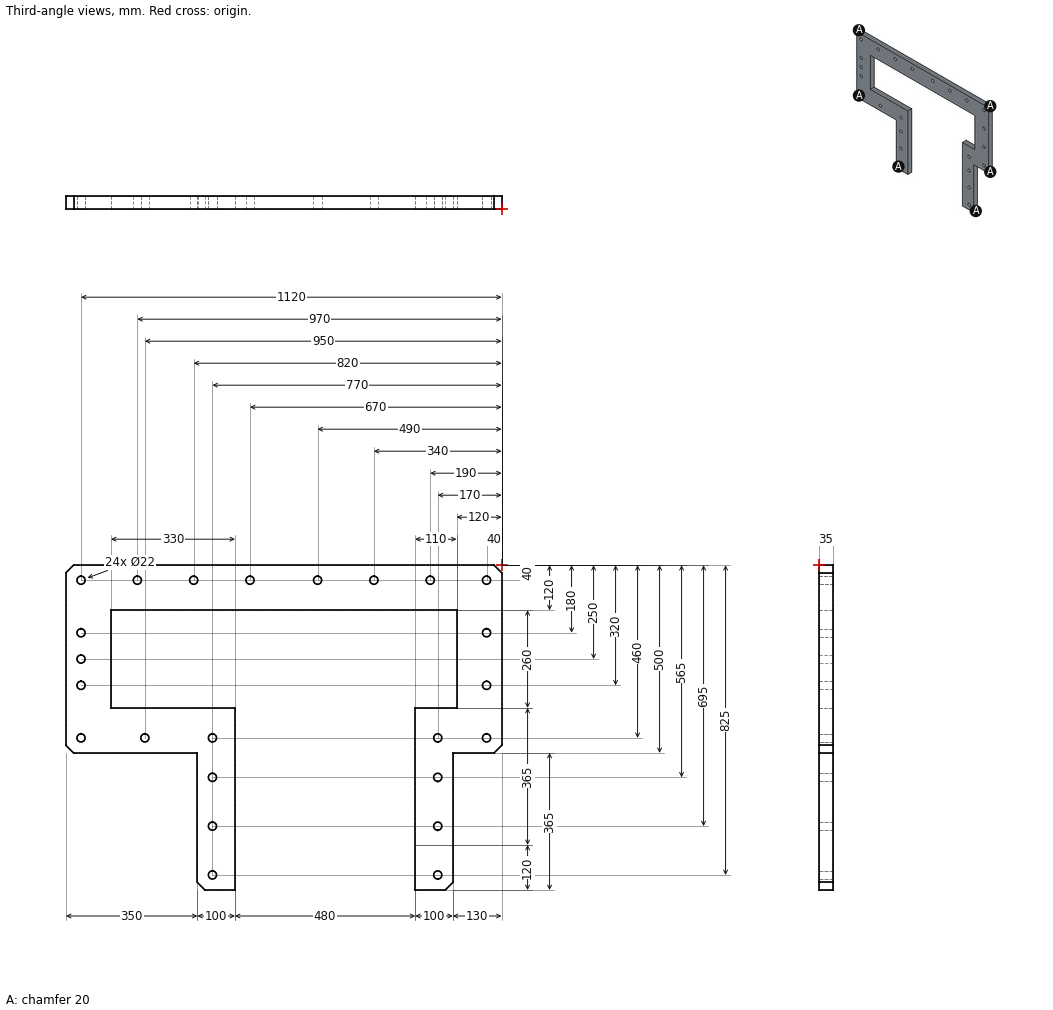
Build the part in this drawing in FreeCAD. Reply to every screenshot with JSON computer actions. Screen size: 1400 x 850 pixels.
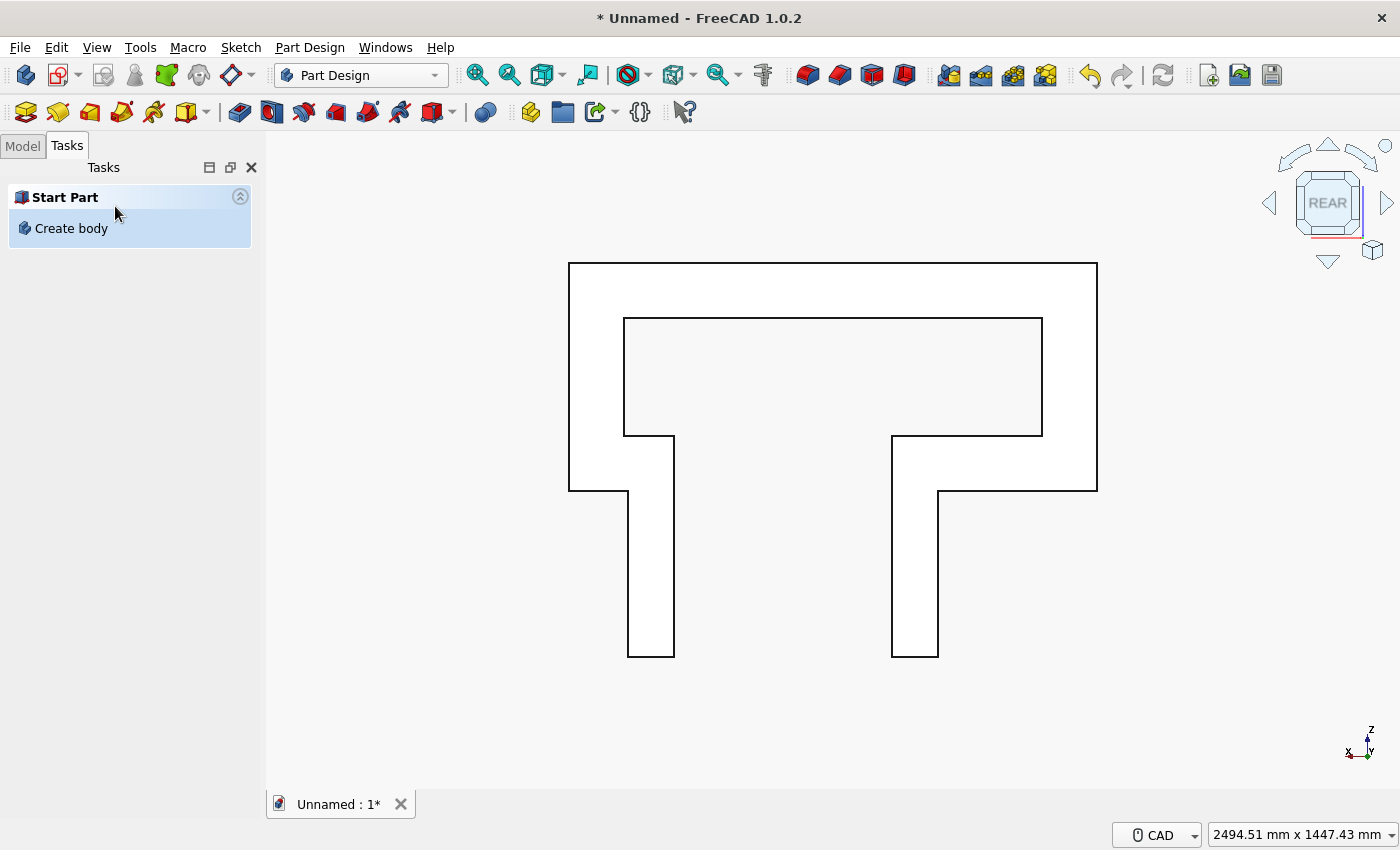
{"action": "scroll", "coordinate": [569, 262], "scroll_direction": "up", "scroll_amount": 5}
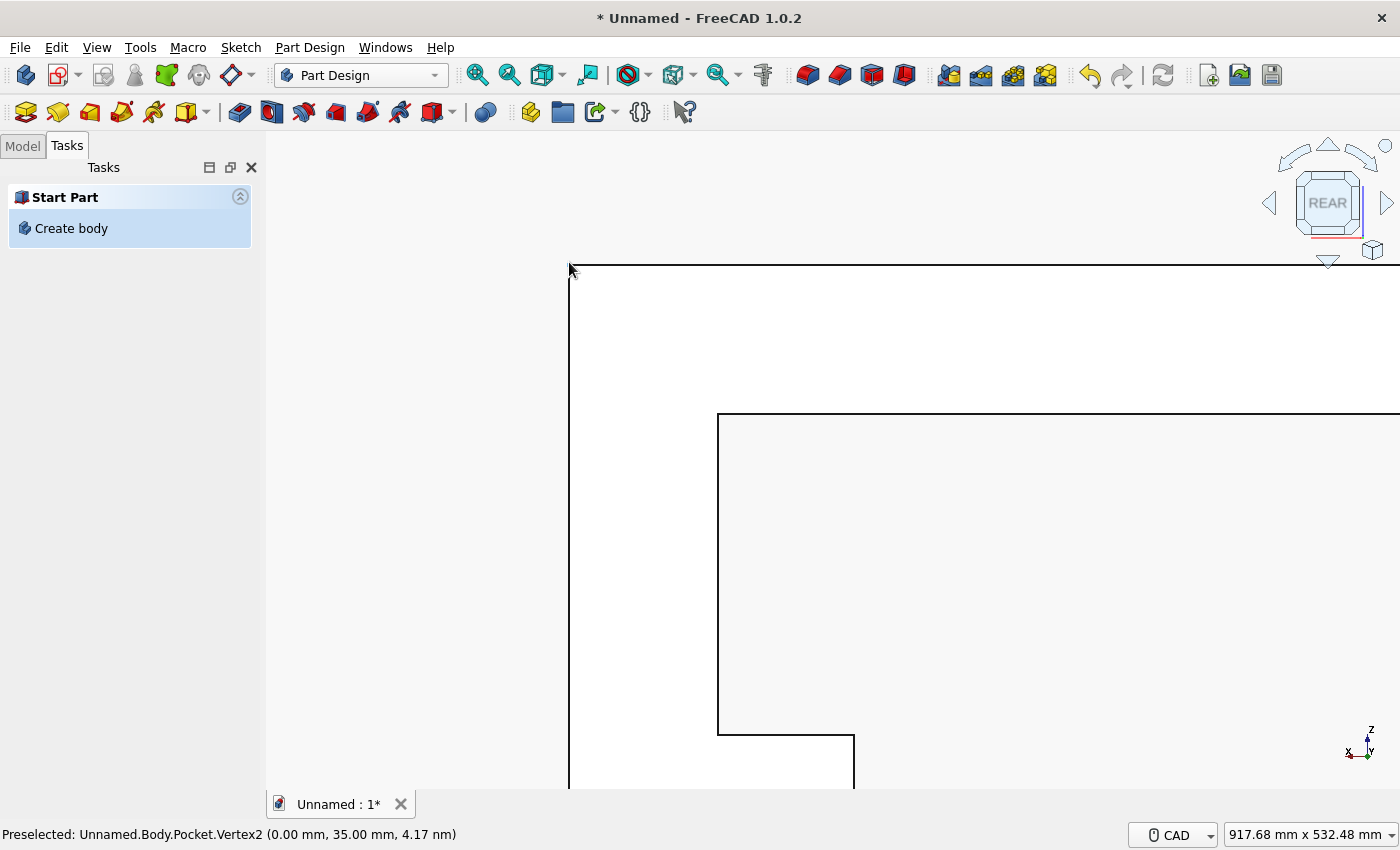
{"action": "left_click", "coordinate": [478, 76]}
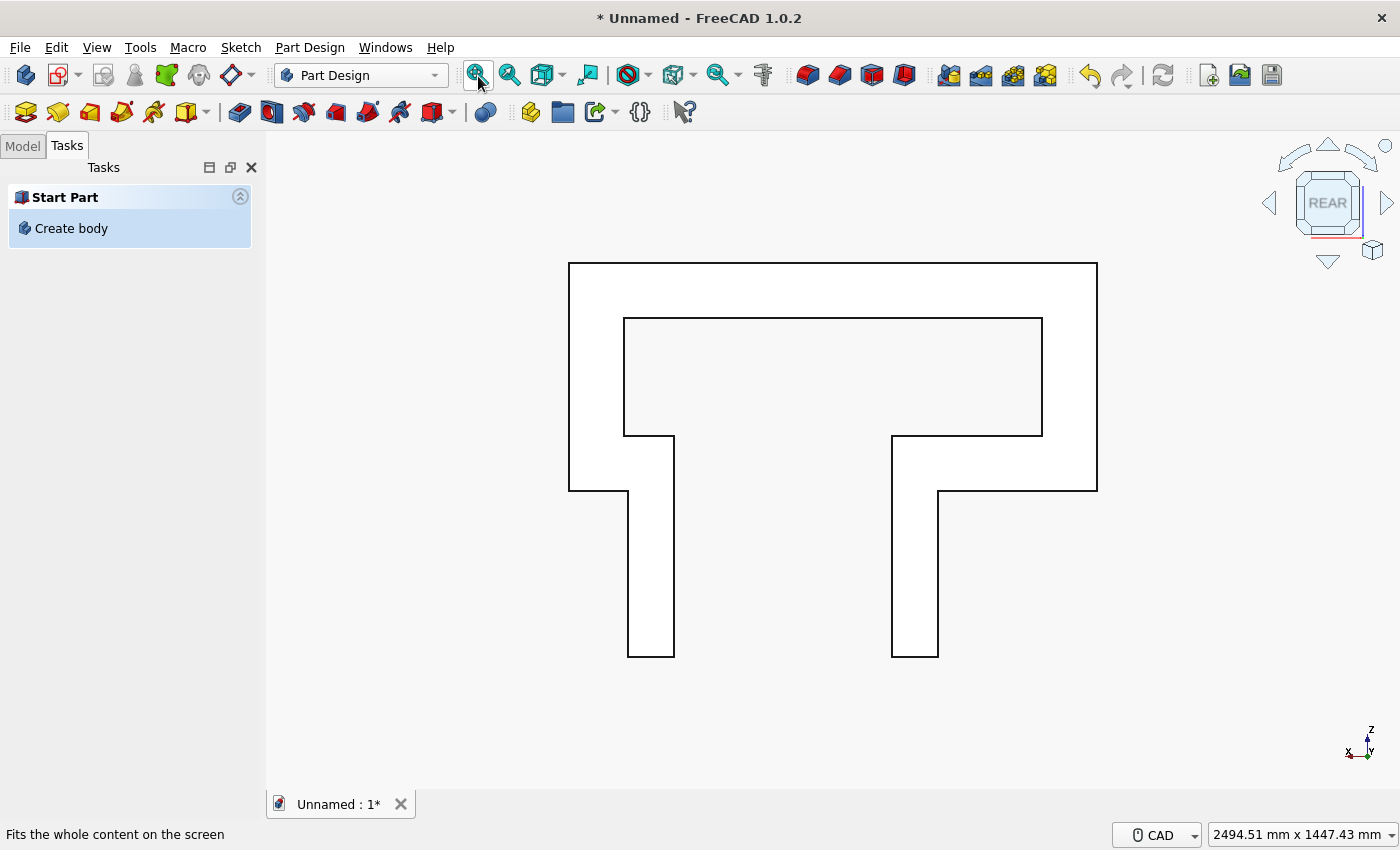
{"action": "key", "text": "0"}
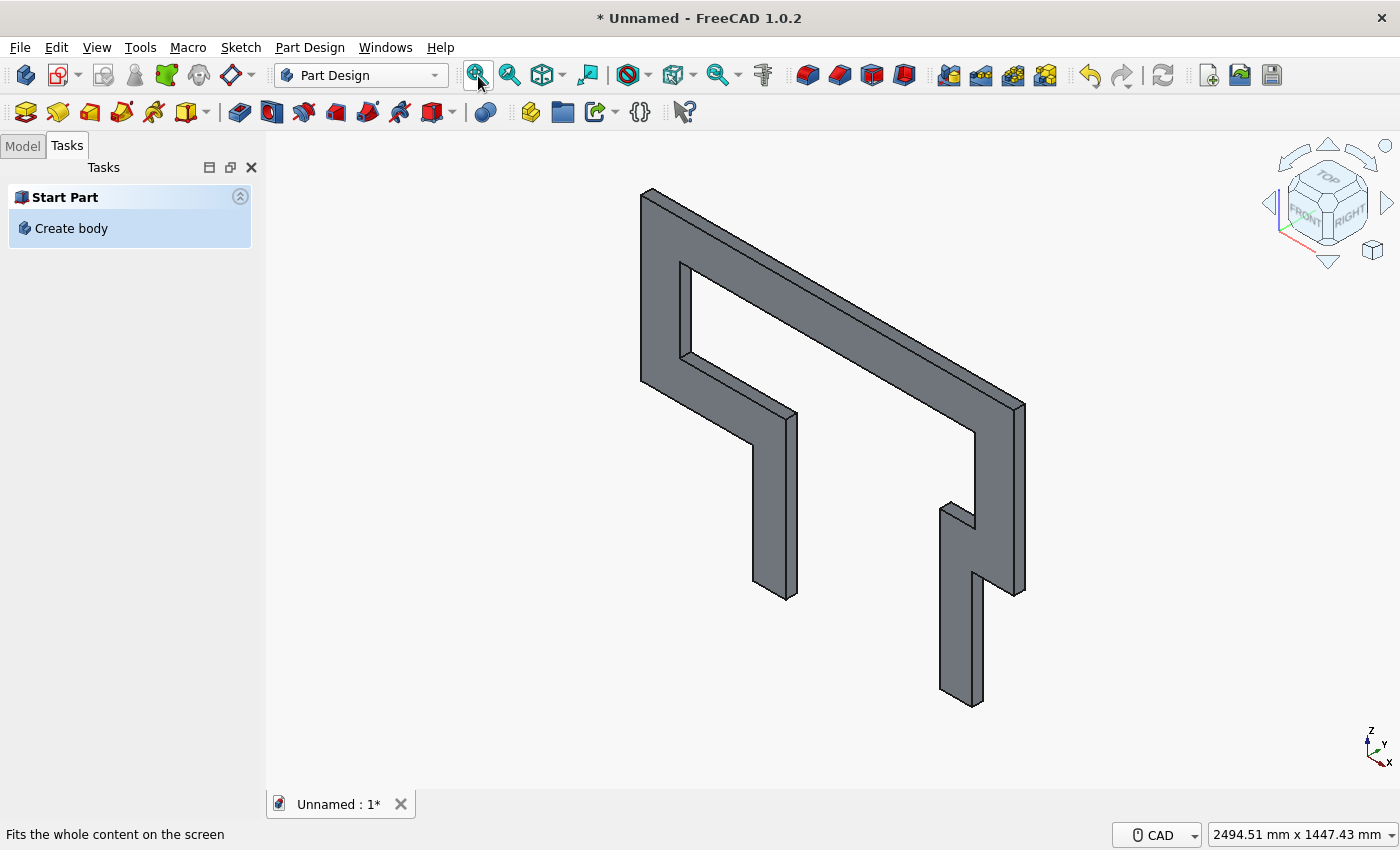
{"action": "left_click", "coordinate": [1021, 405]}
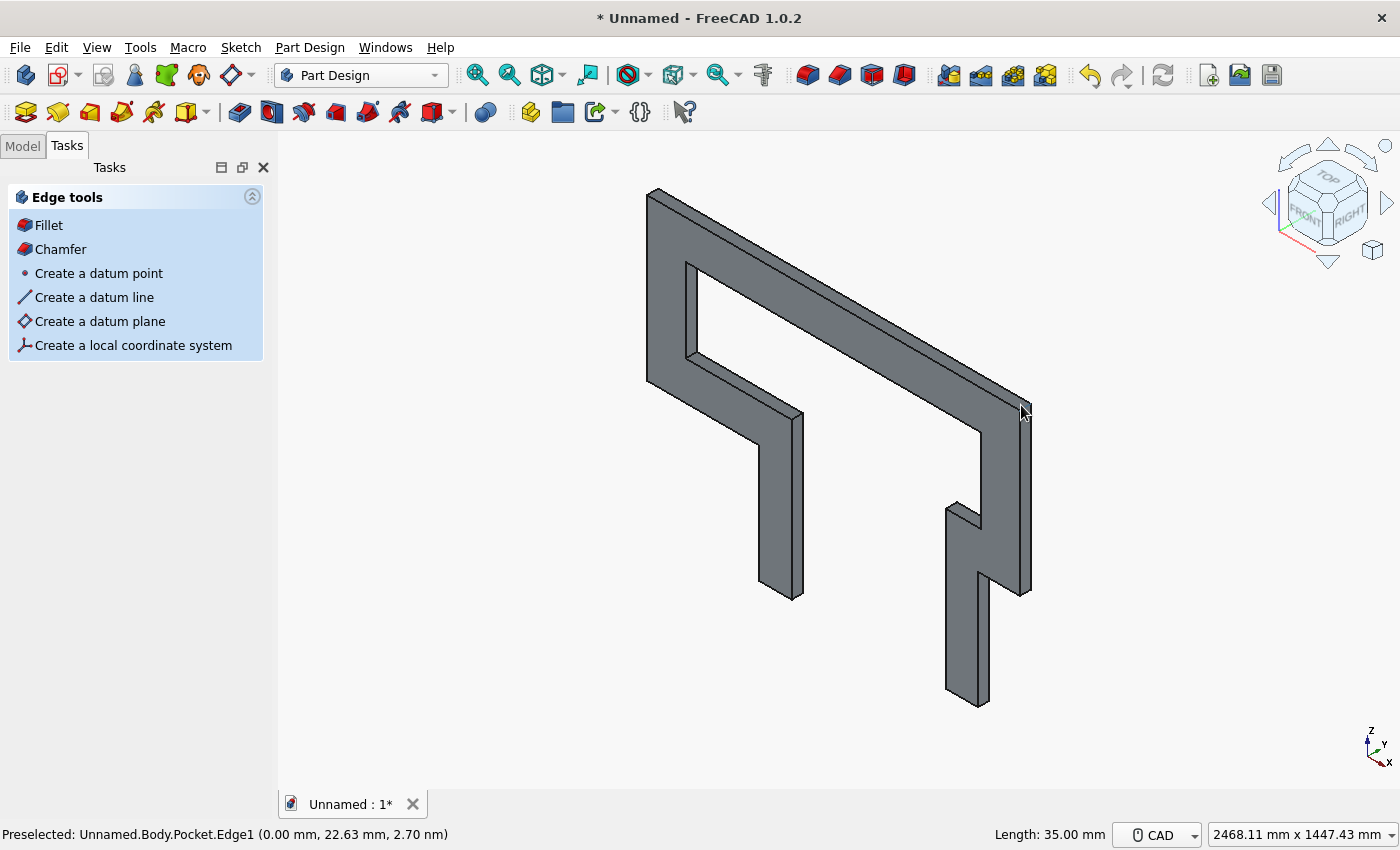
{"action": "scroll", "coordinate": [653, 191], "scroll_direction": "up", "scroll_amount": 5}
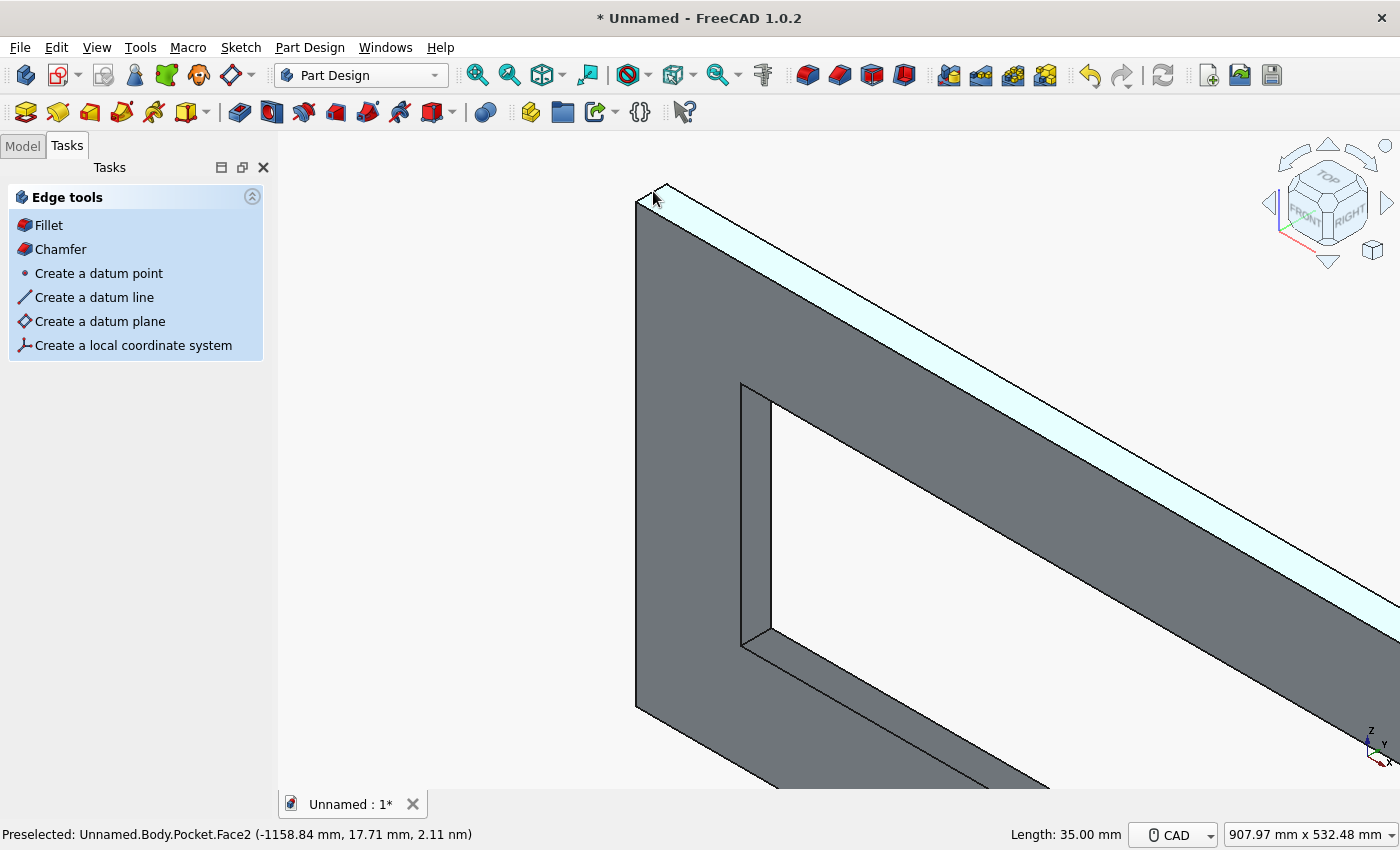
{"action": "key", "text": "v f"}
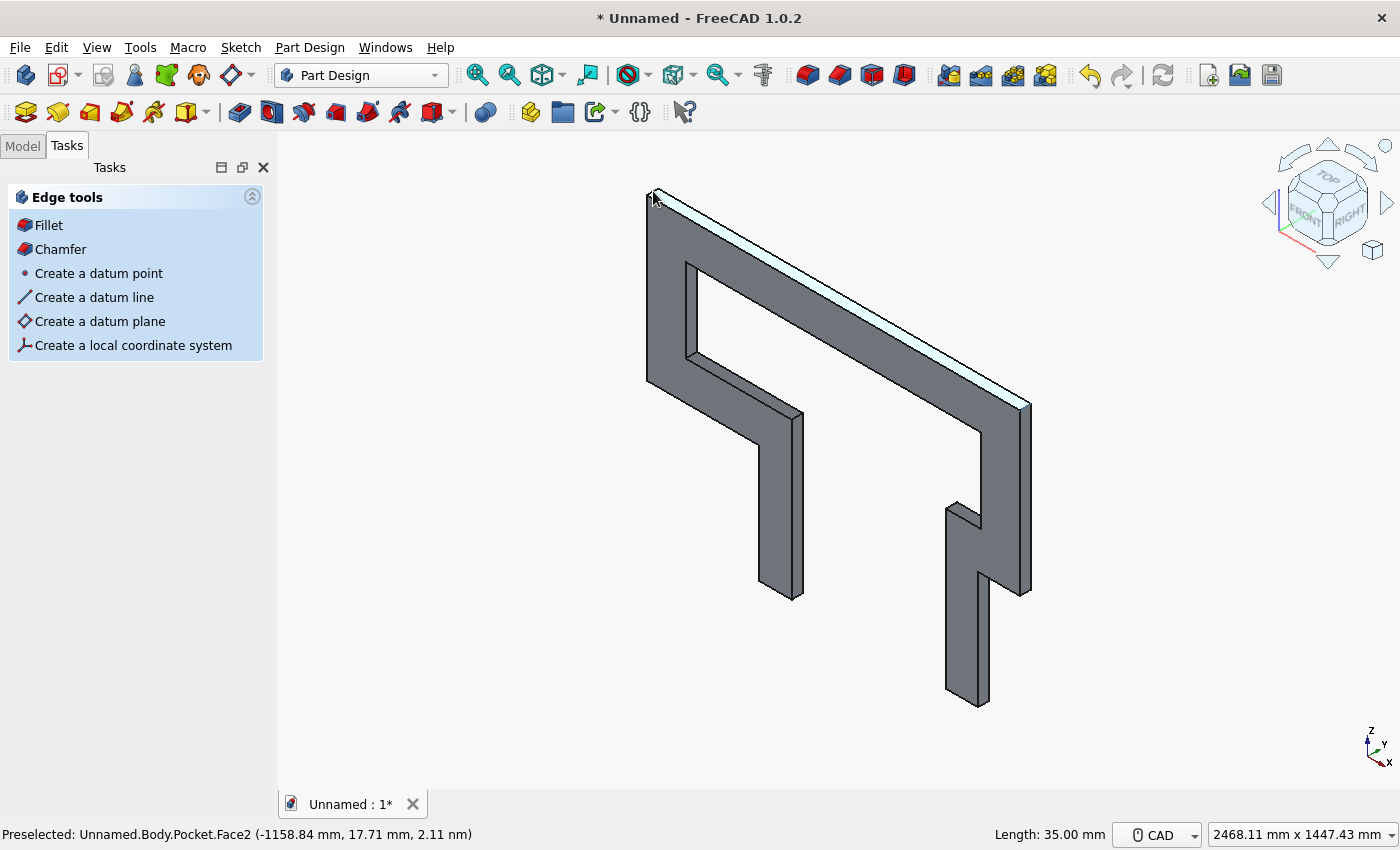
{"action": "key", "text": "2"}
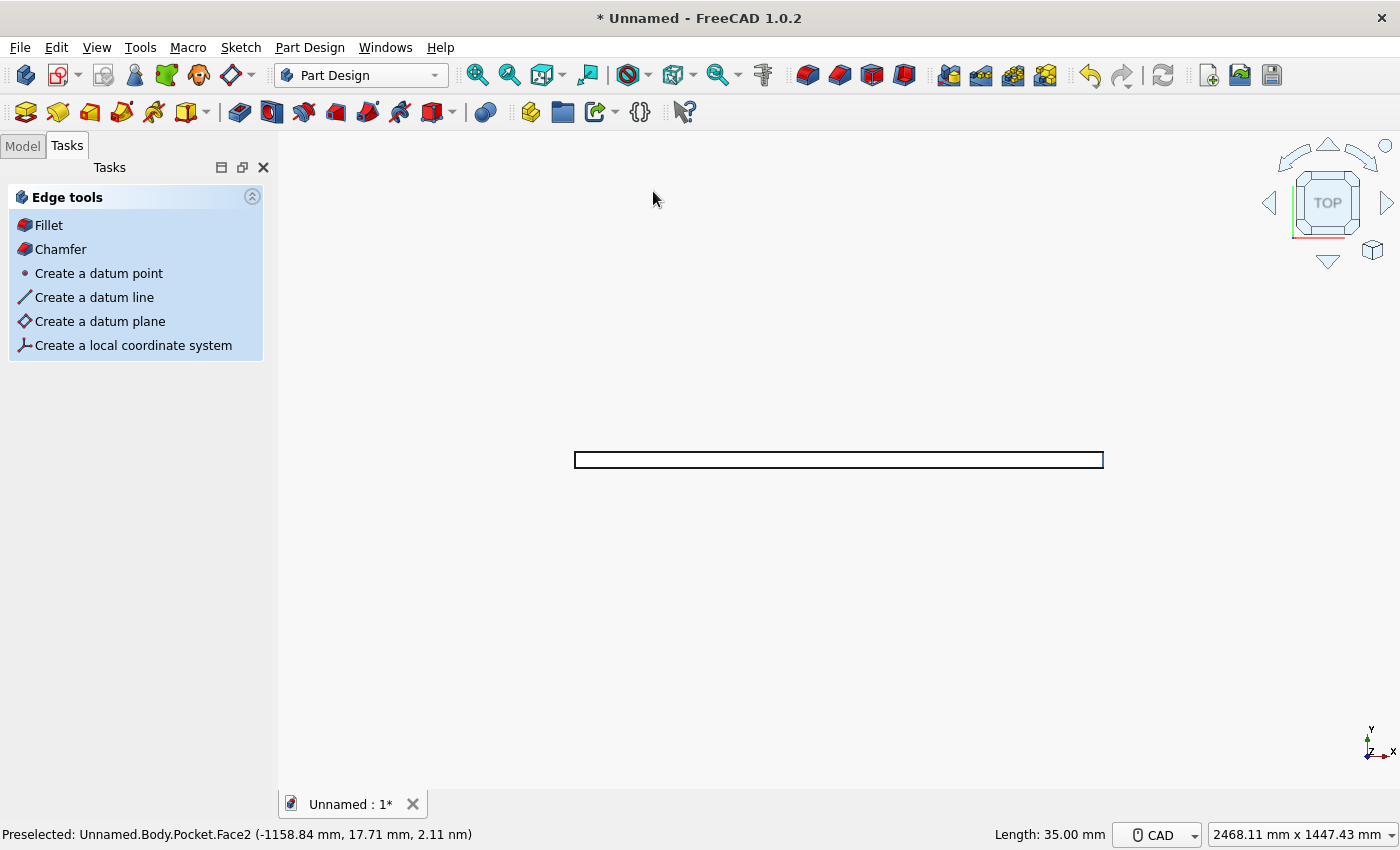
{"action": "left_click", "coordinate": [575, 459], "text": "ctrl"}